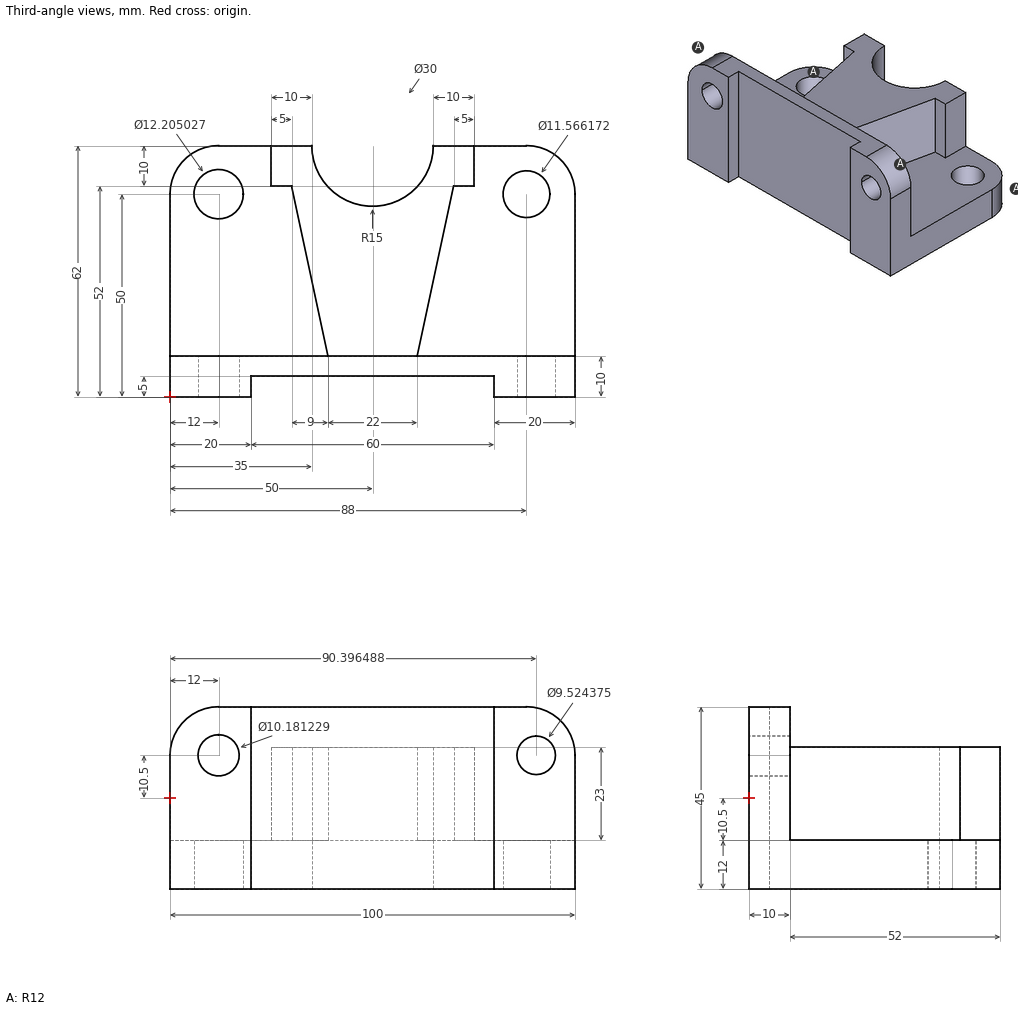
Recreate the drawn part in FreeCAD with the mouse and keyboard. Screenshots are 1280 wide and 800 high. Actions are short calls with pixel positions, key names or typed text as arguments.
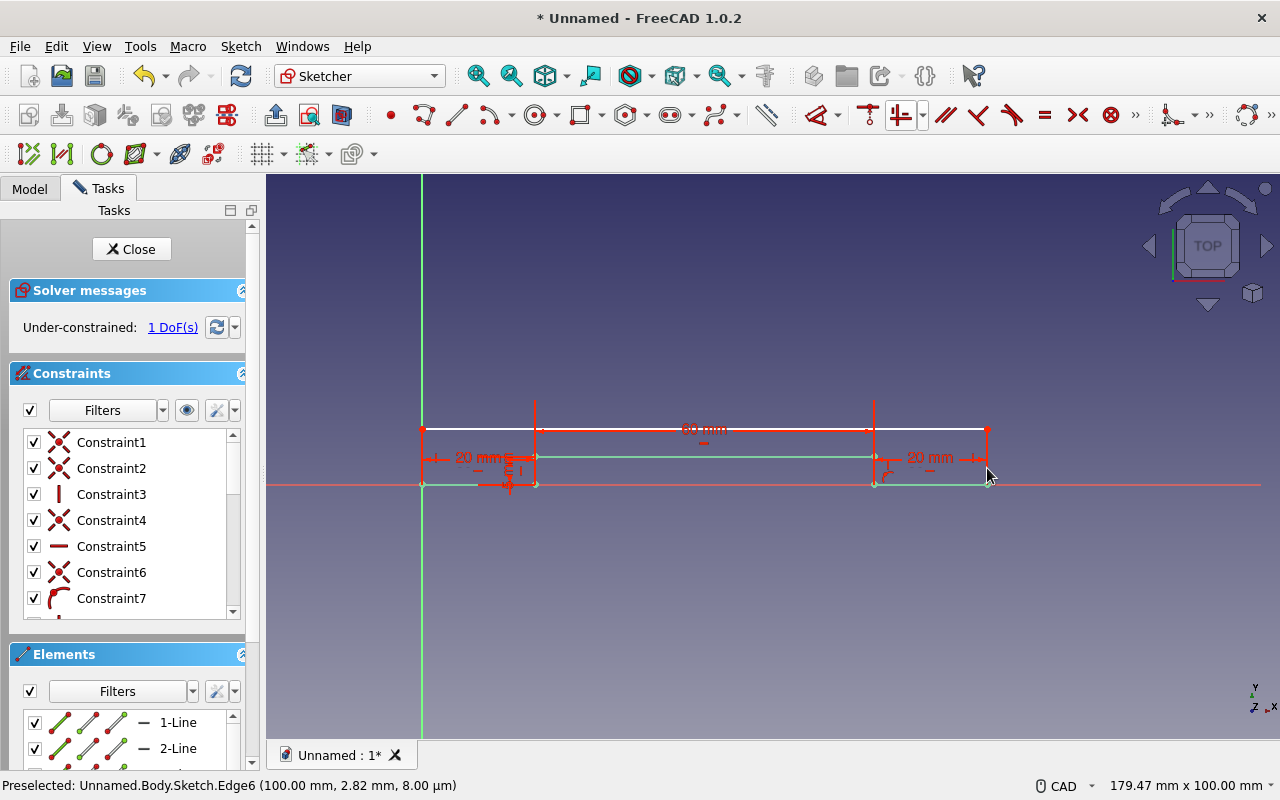
key(i)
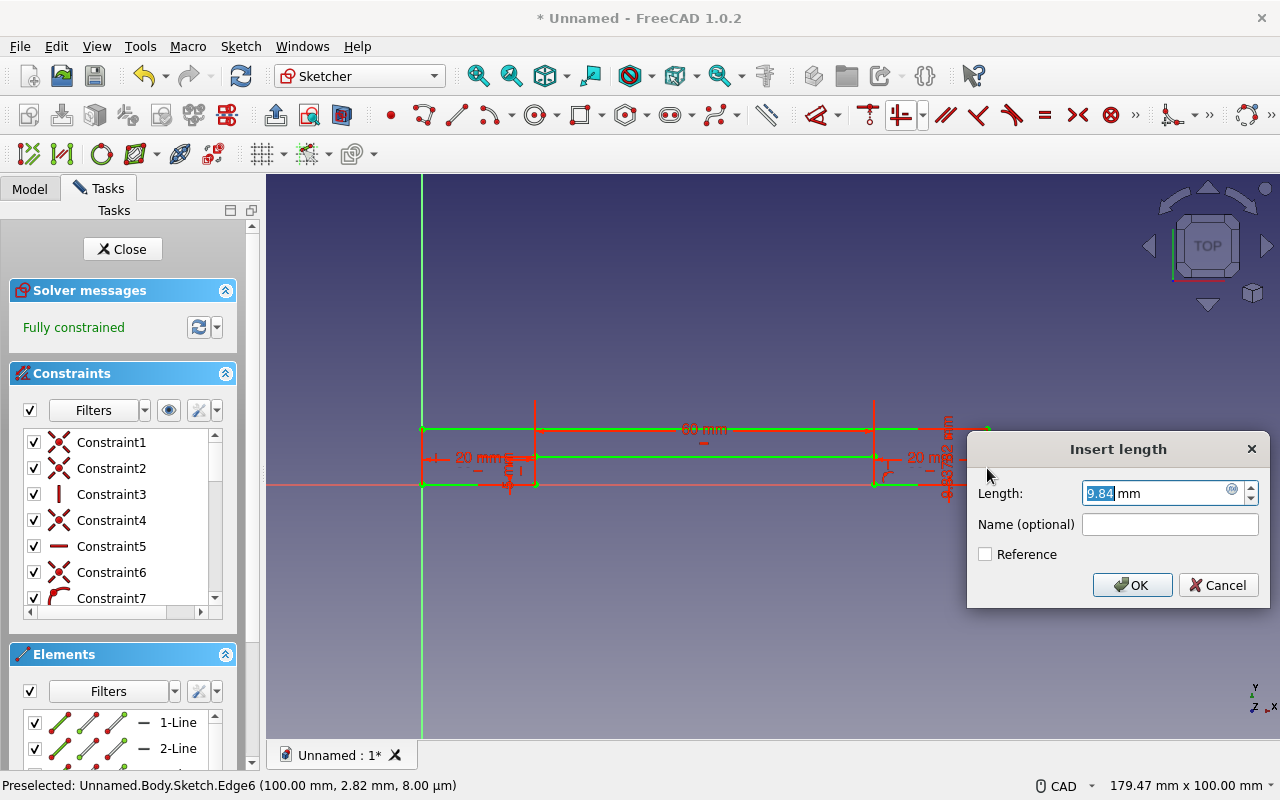
text(10)
key(Return)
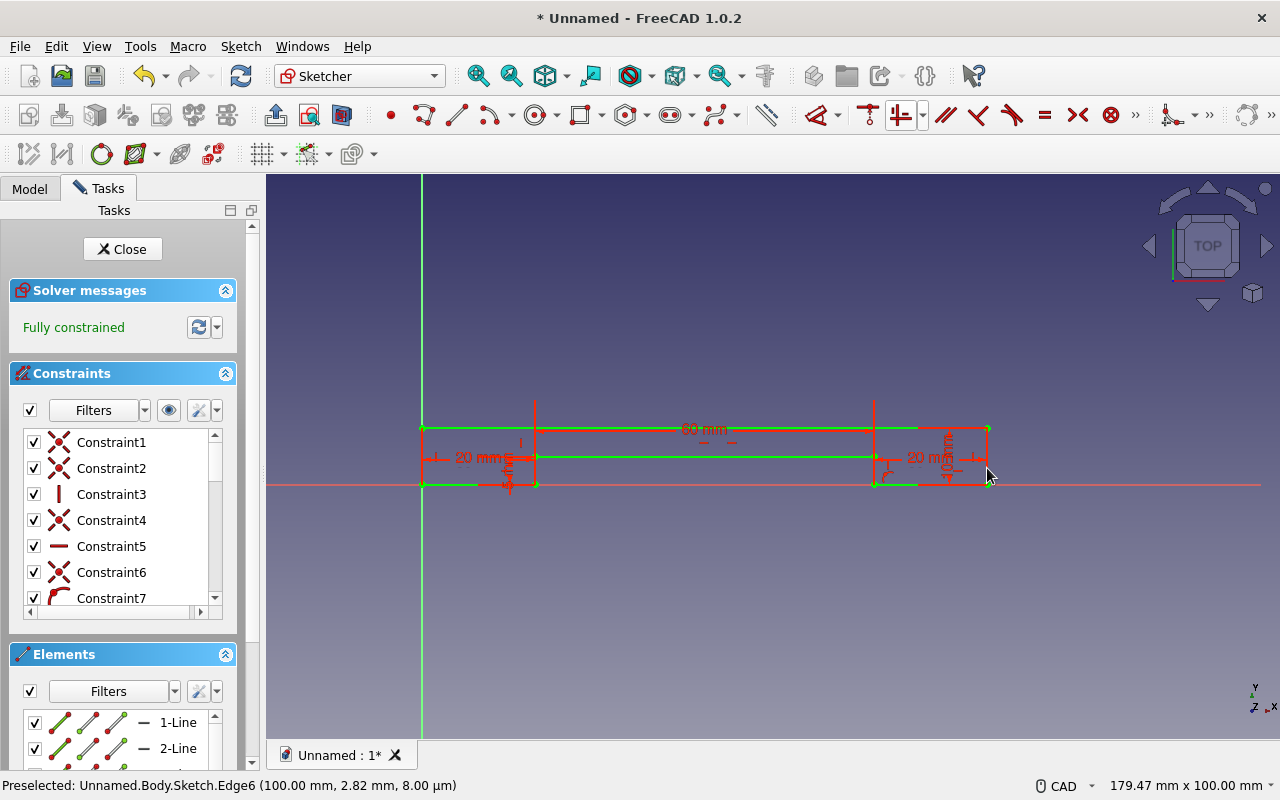
click(123, 249)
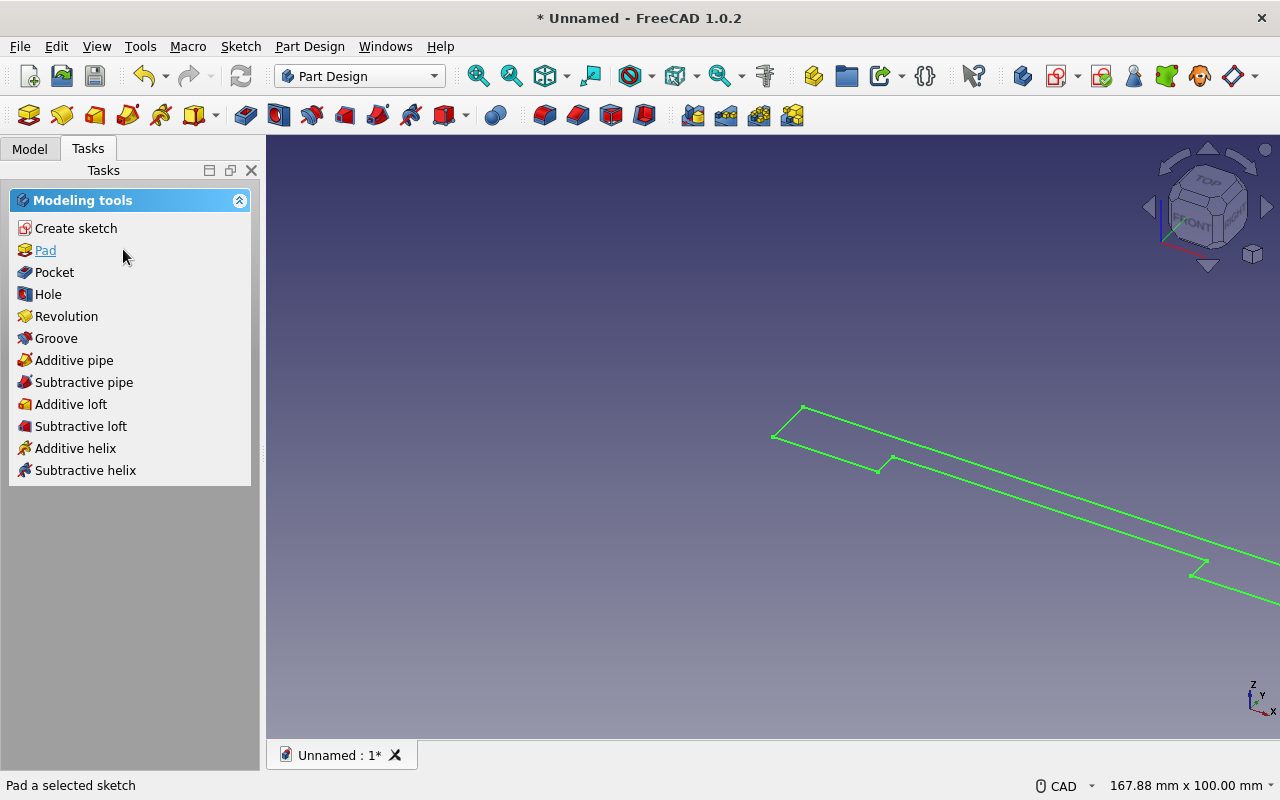
click(29, 116)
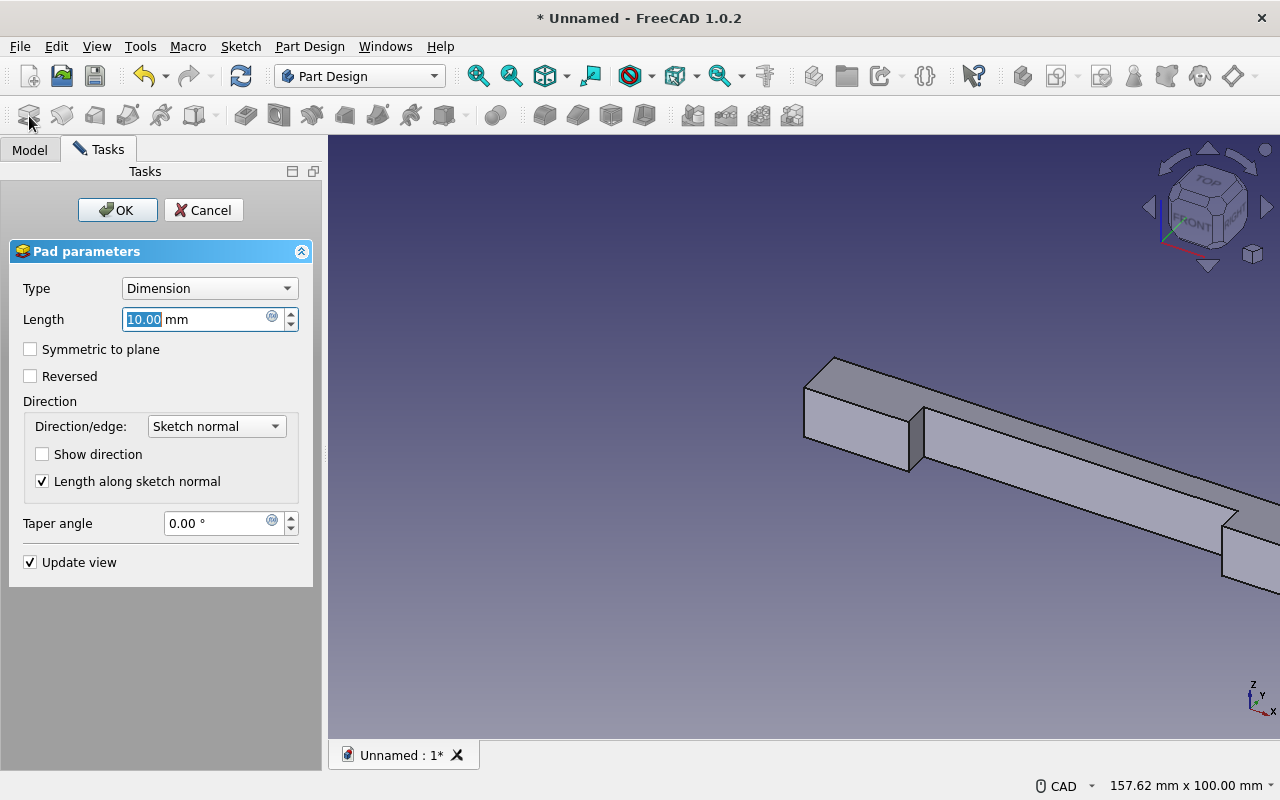
text(45)
key(Tab)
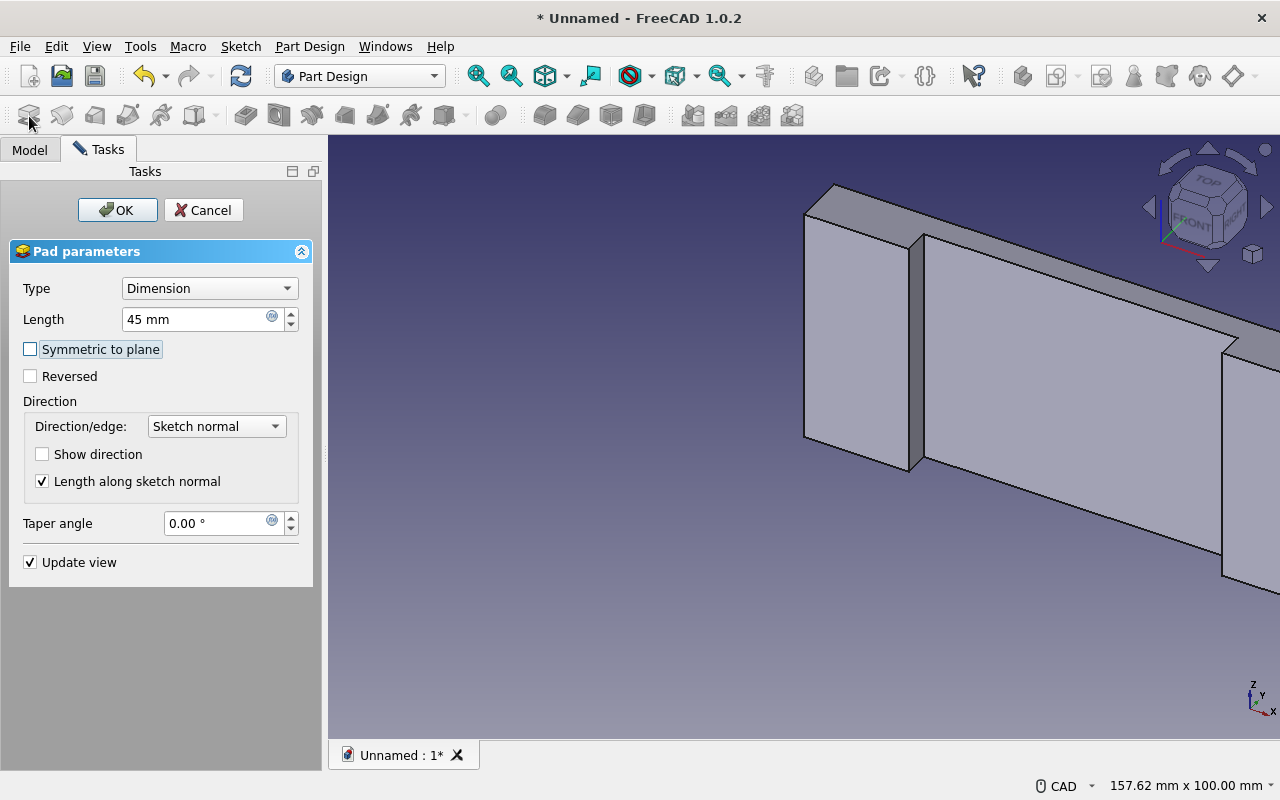
click(31, 349)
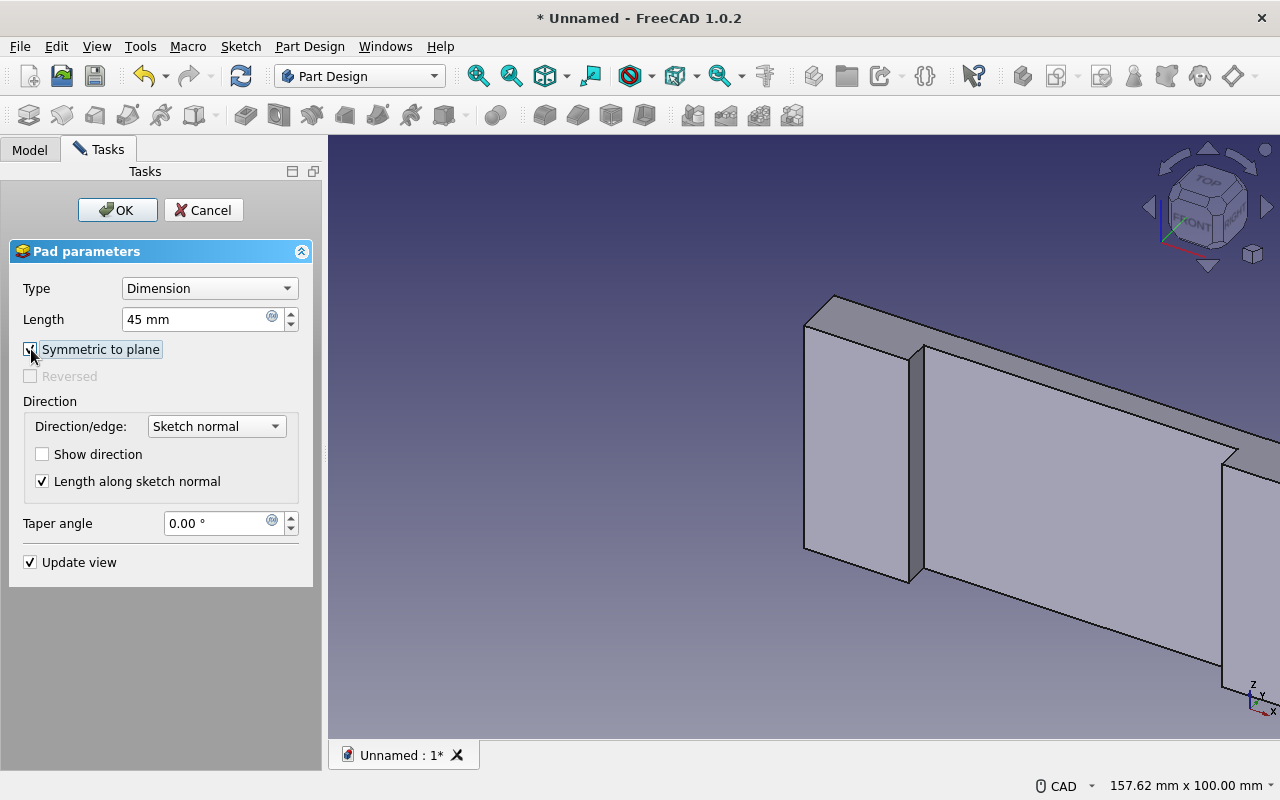
click(118, 210)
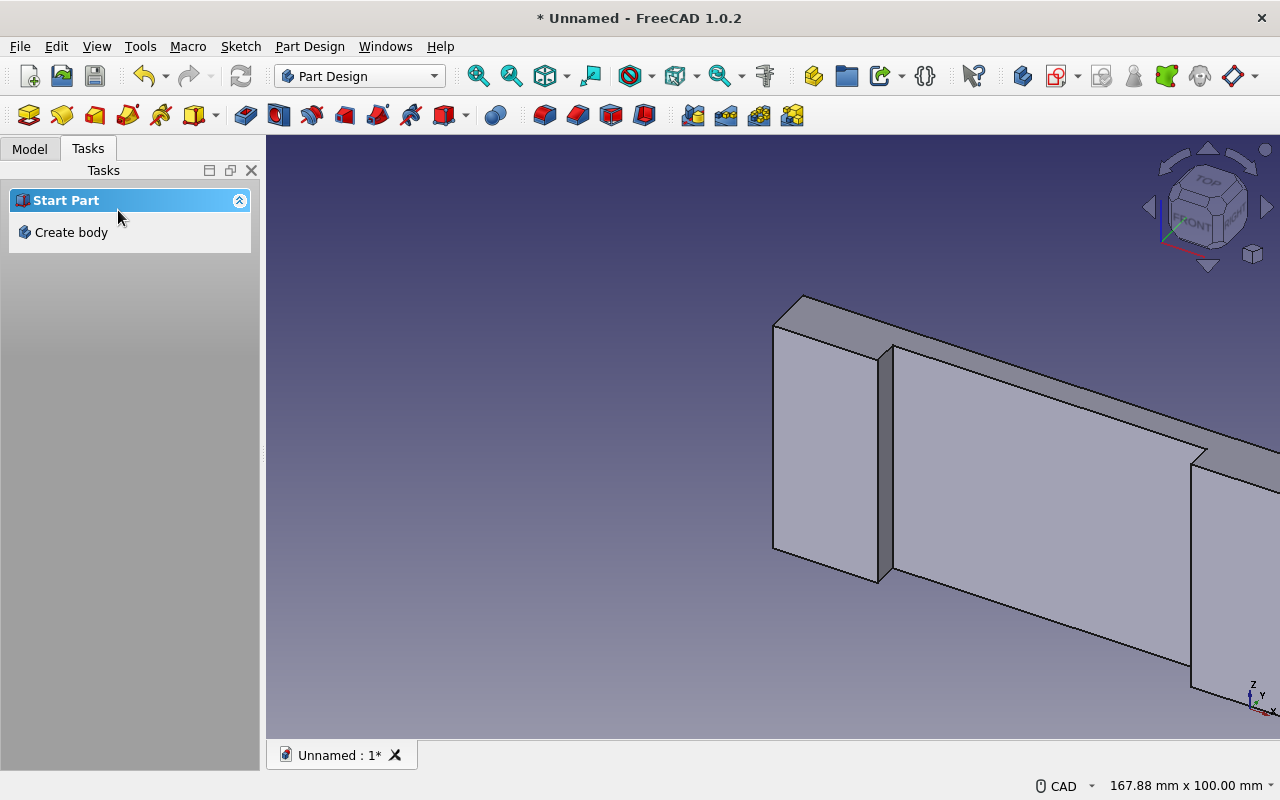
key(v)
key(f)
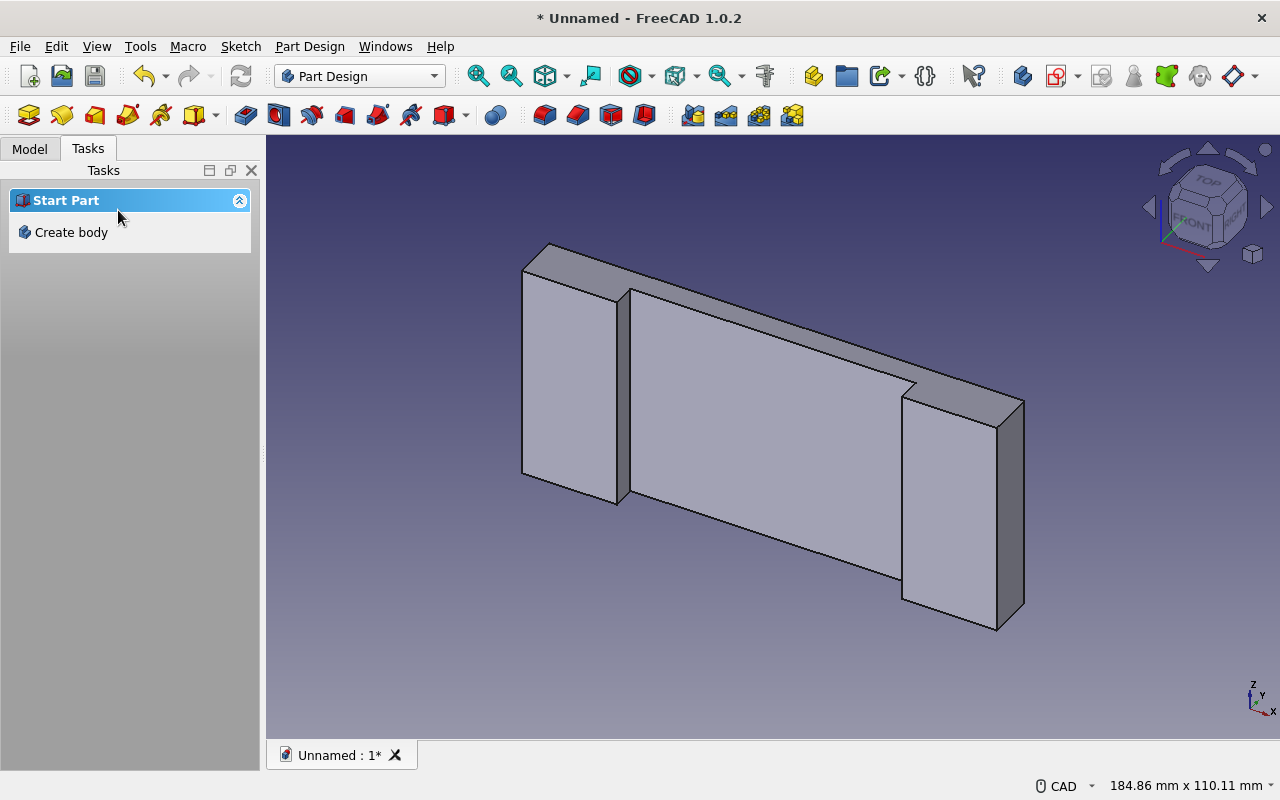
click(1011, 457)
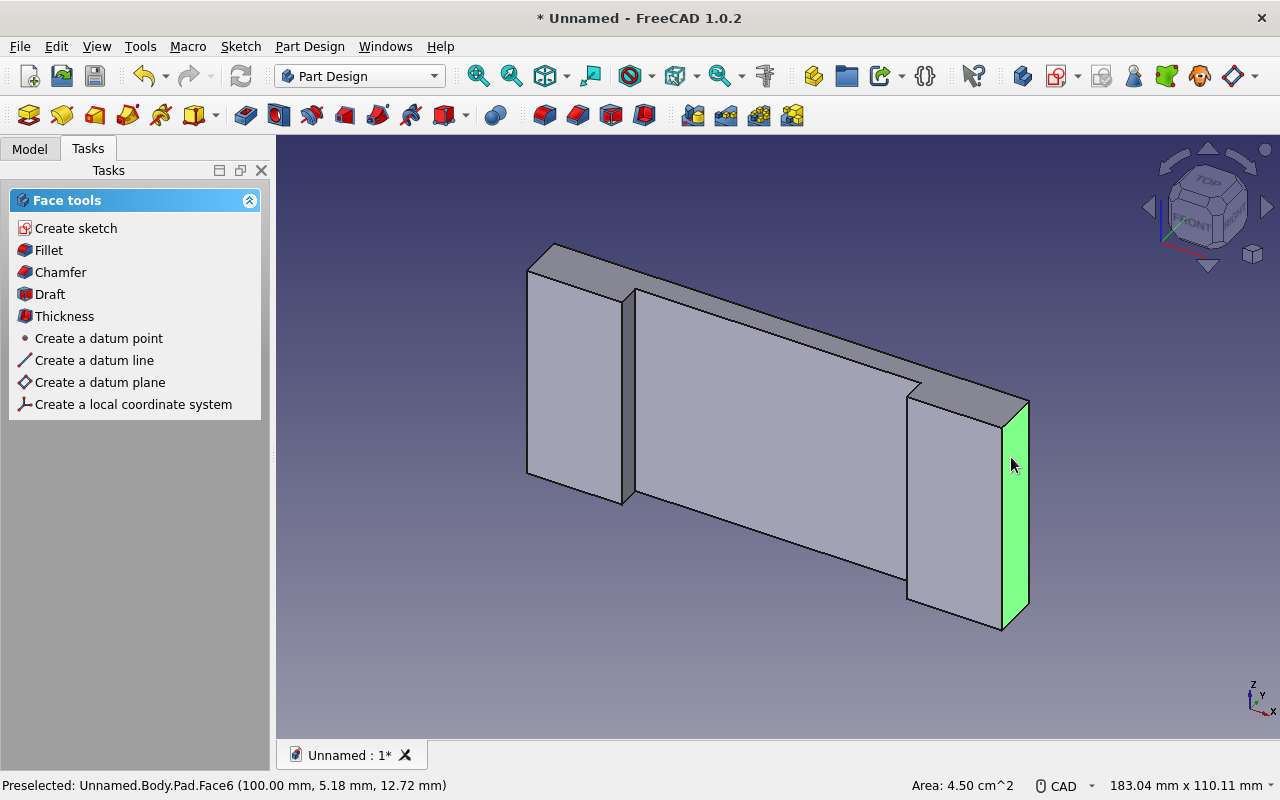
click(1056, 76)